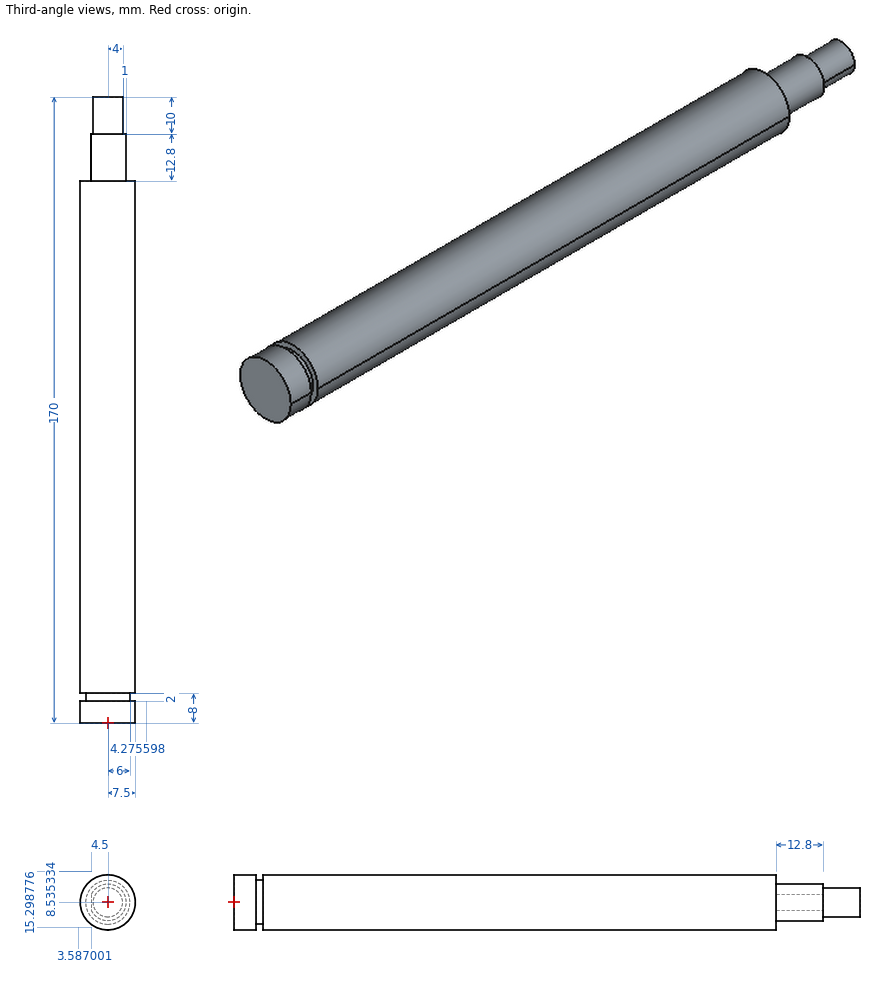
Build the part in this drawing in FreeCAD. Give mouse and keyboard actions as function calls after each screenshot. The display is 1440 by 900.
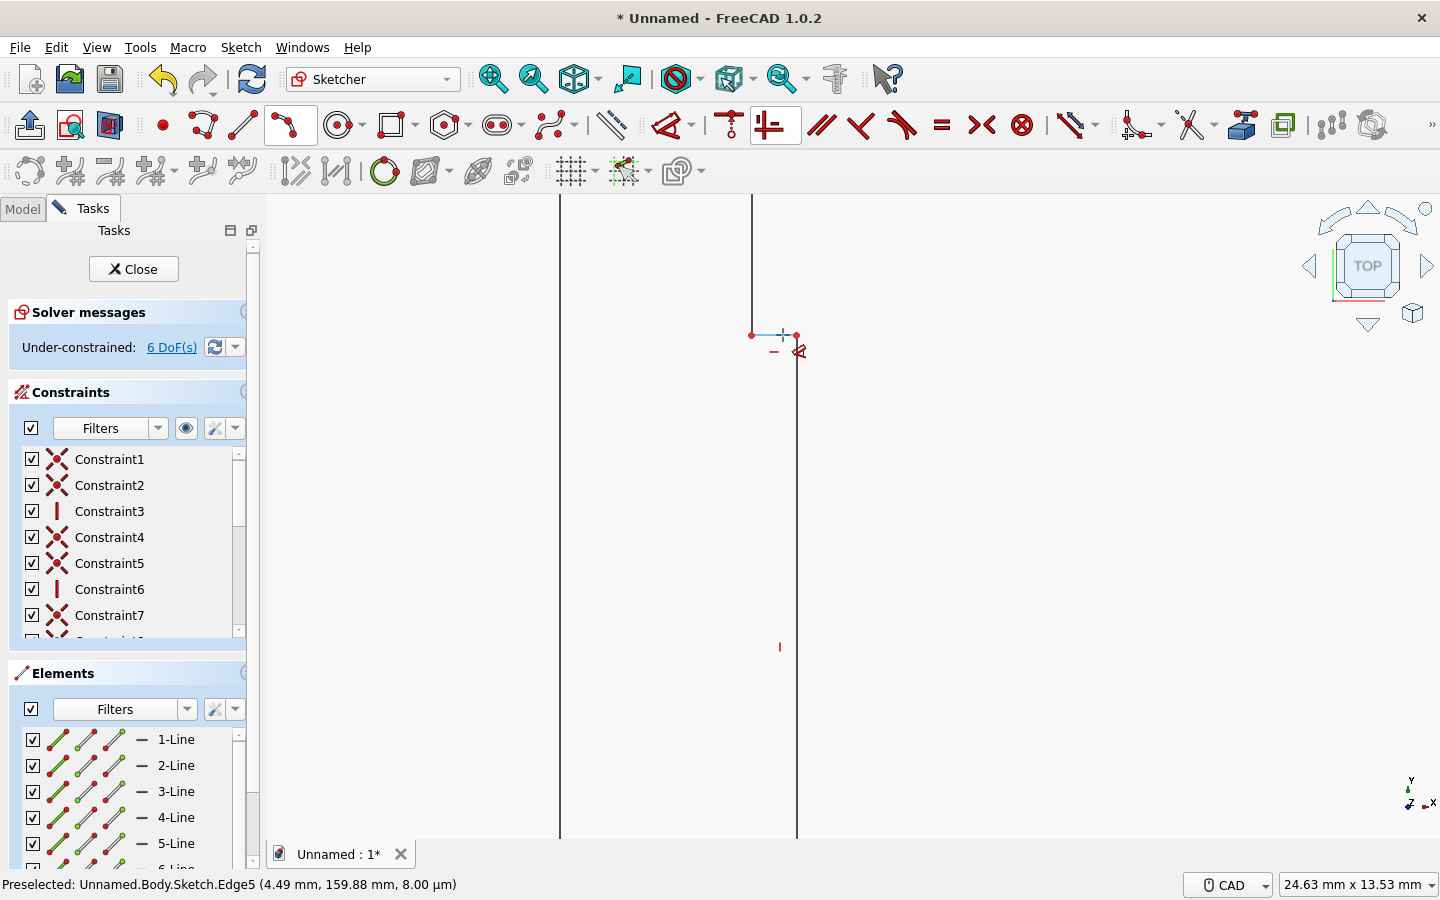
click(783, 335)
click(774, 301)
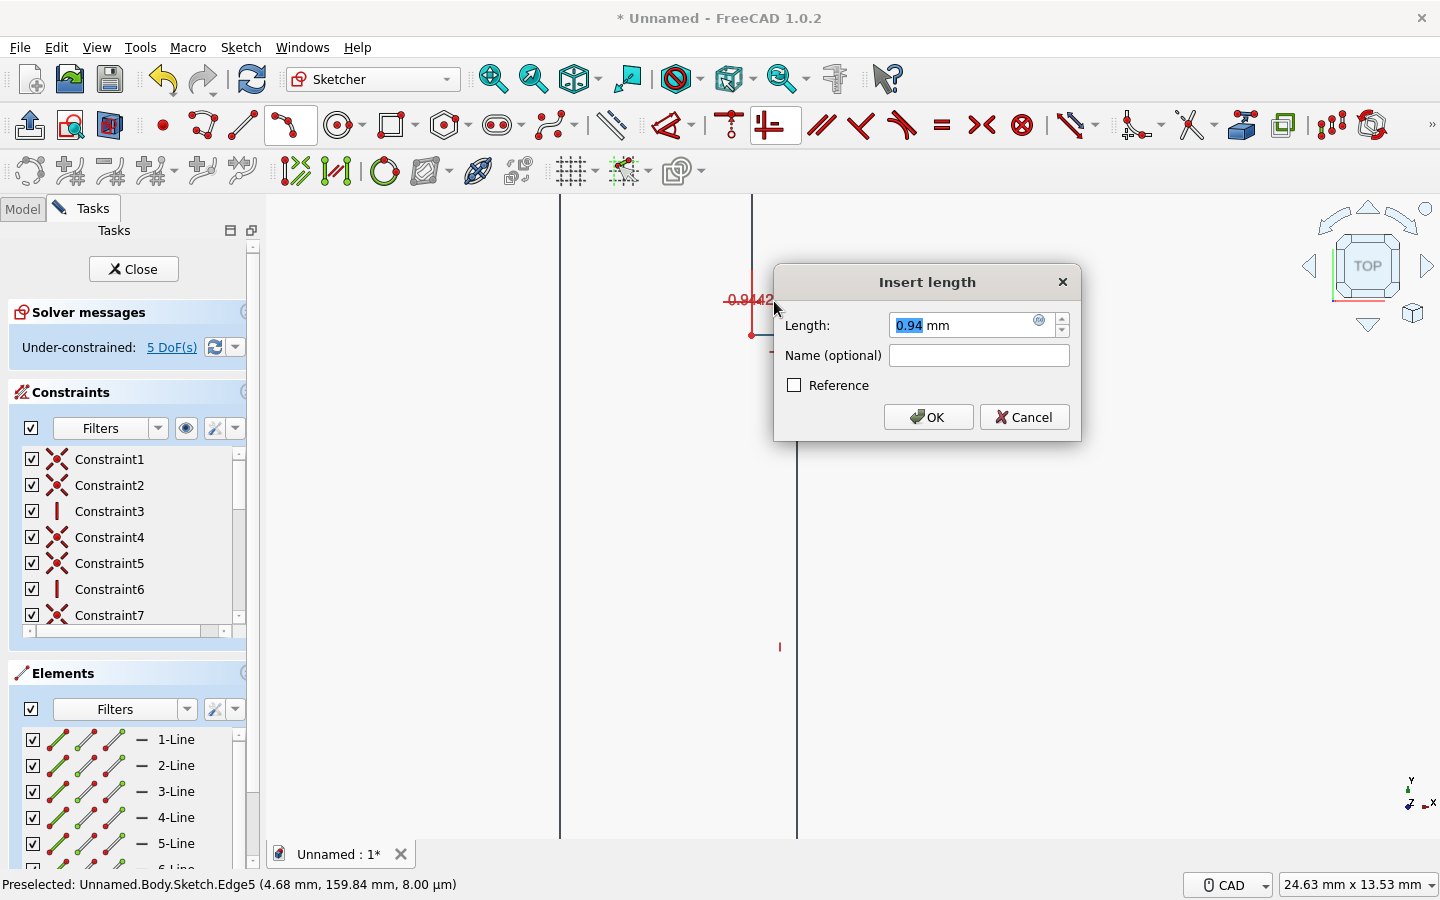
text(1)
key(Return)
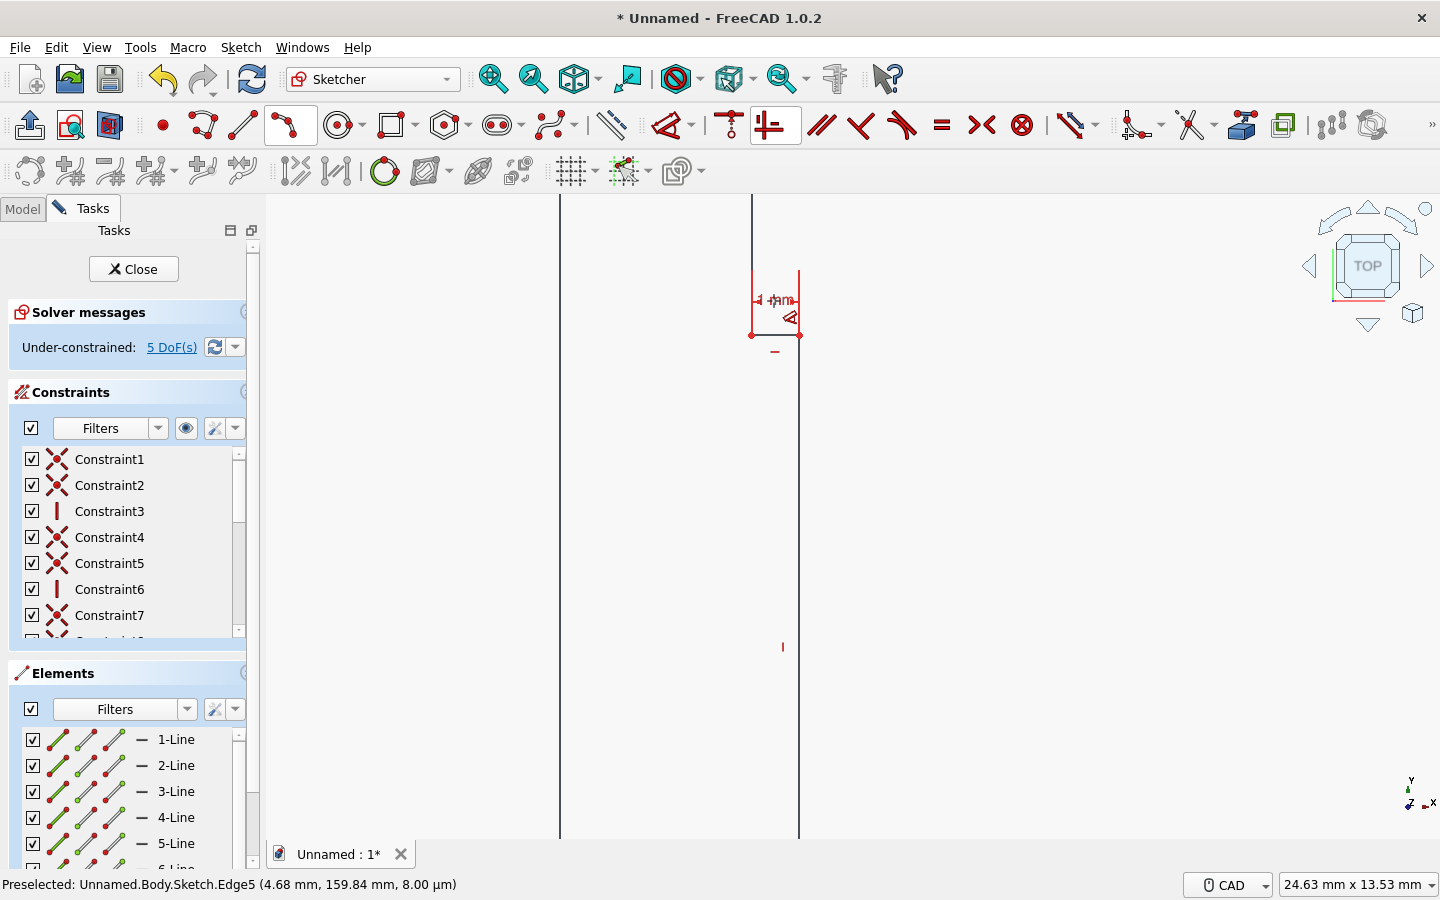
scroll(787, 339, down, 15)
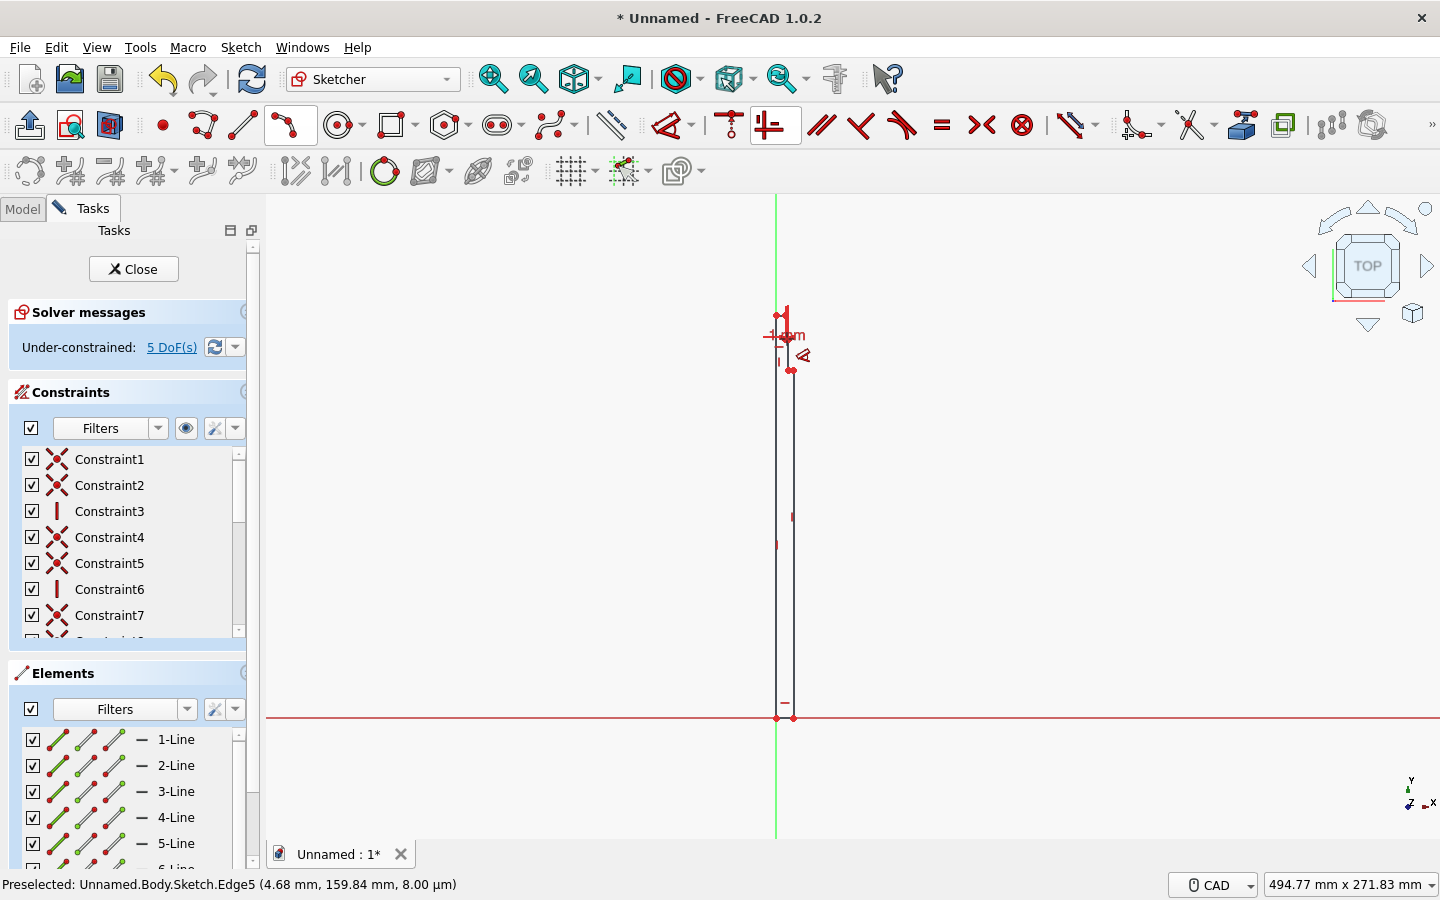
scroll(783, 316, up, 8)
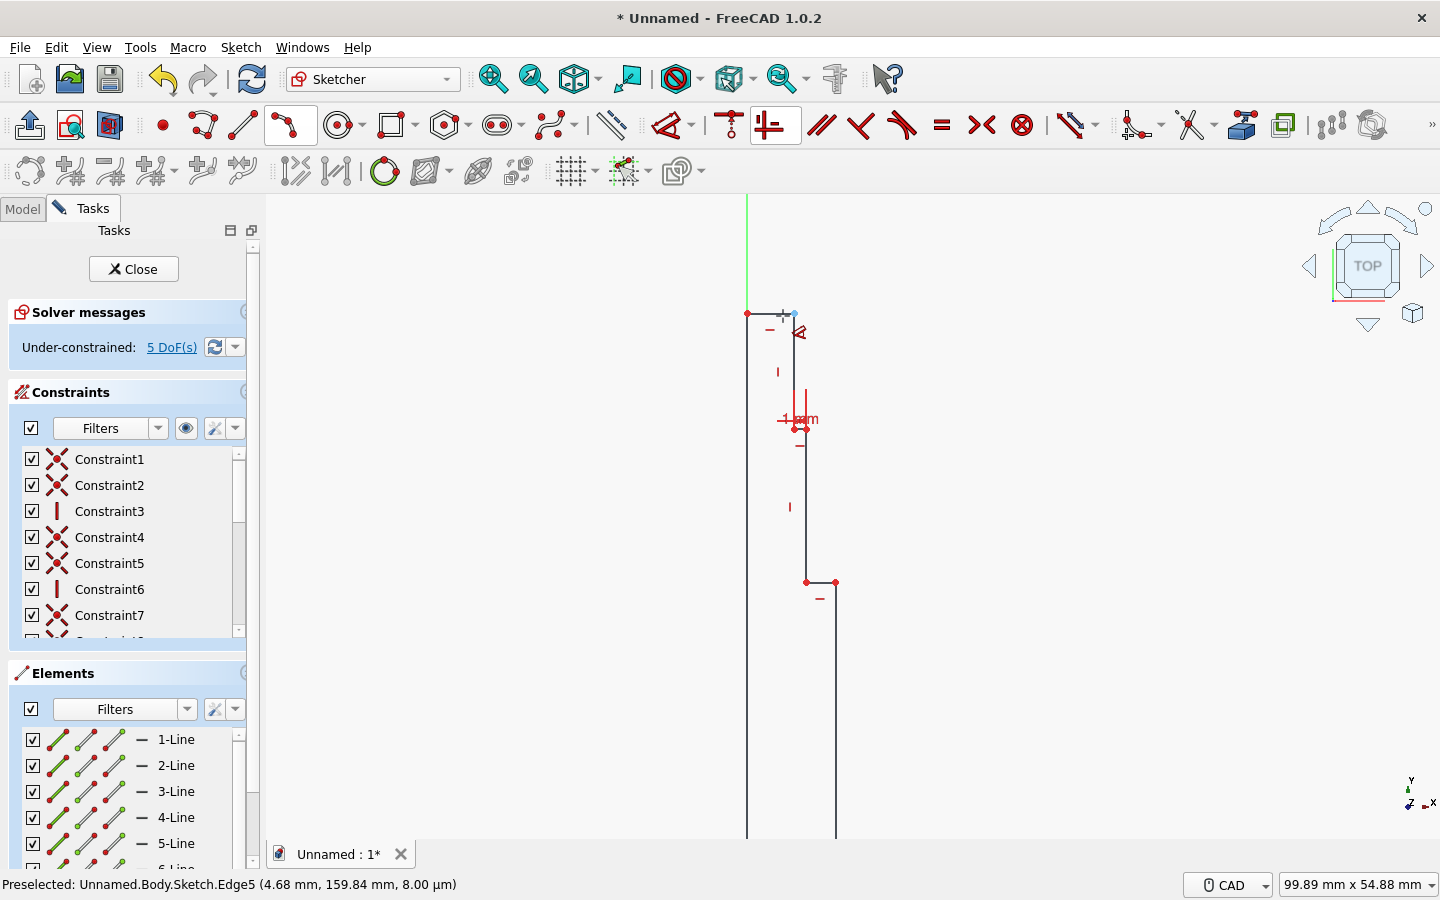
click(780, 314)
click(771, 280)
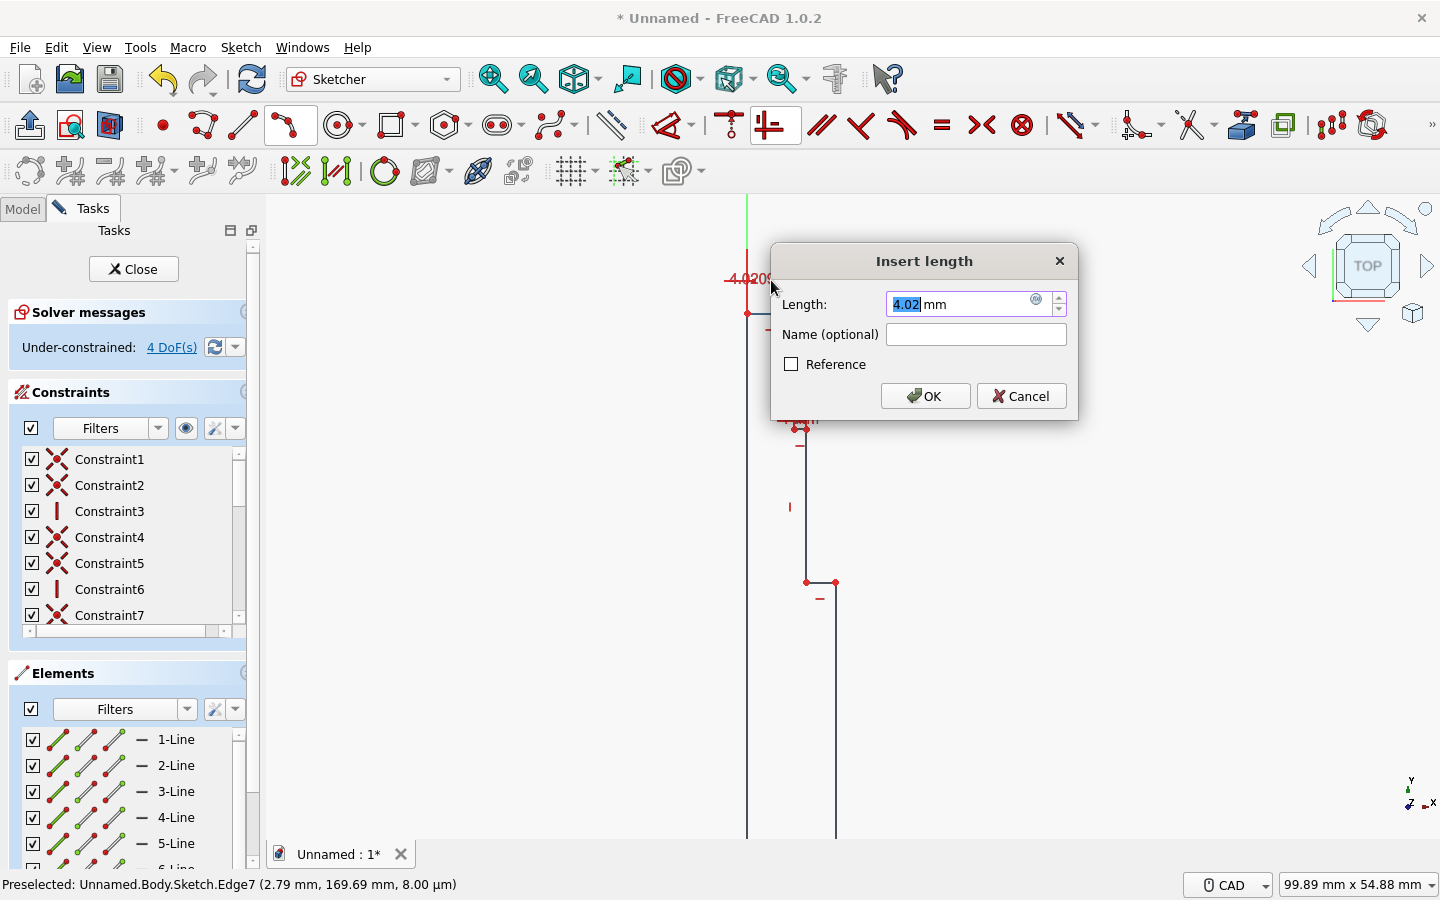
text(4)
key(Return)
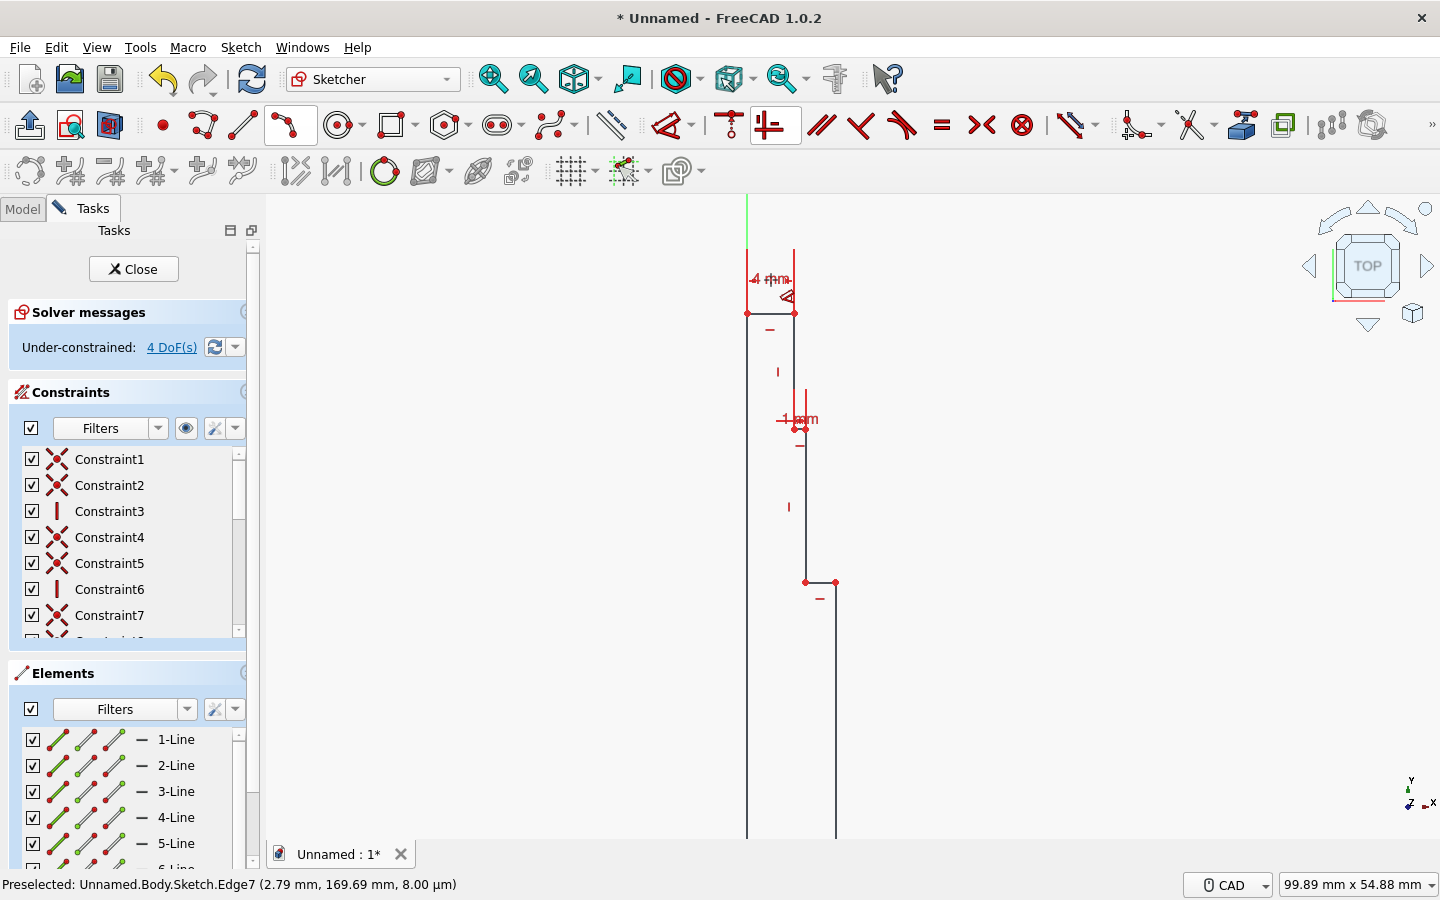
click(794, 395)
click(828, 371)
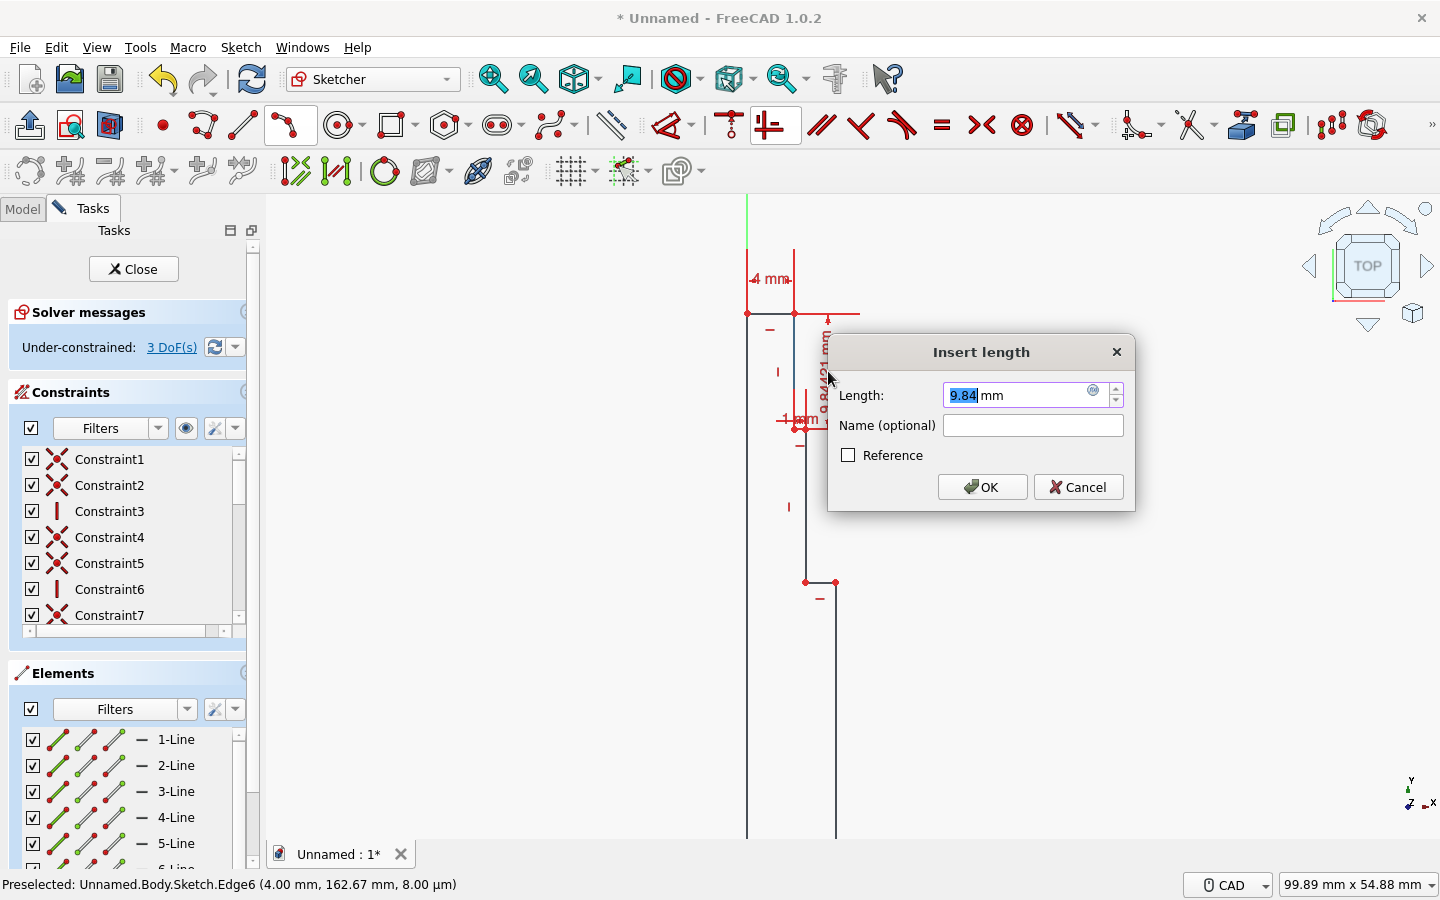
text(10)
key(Return)